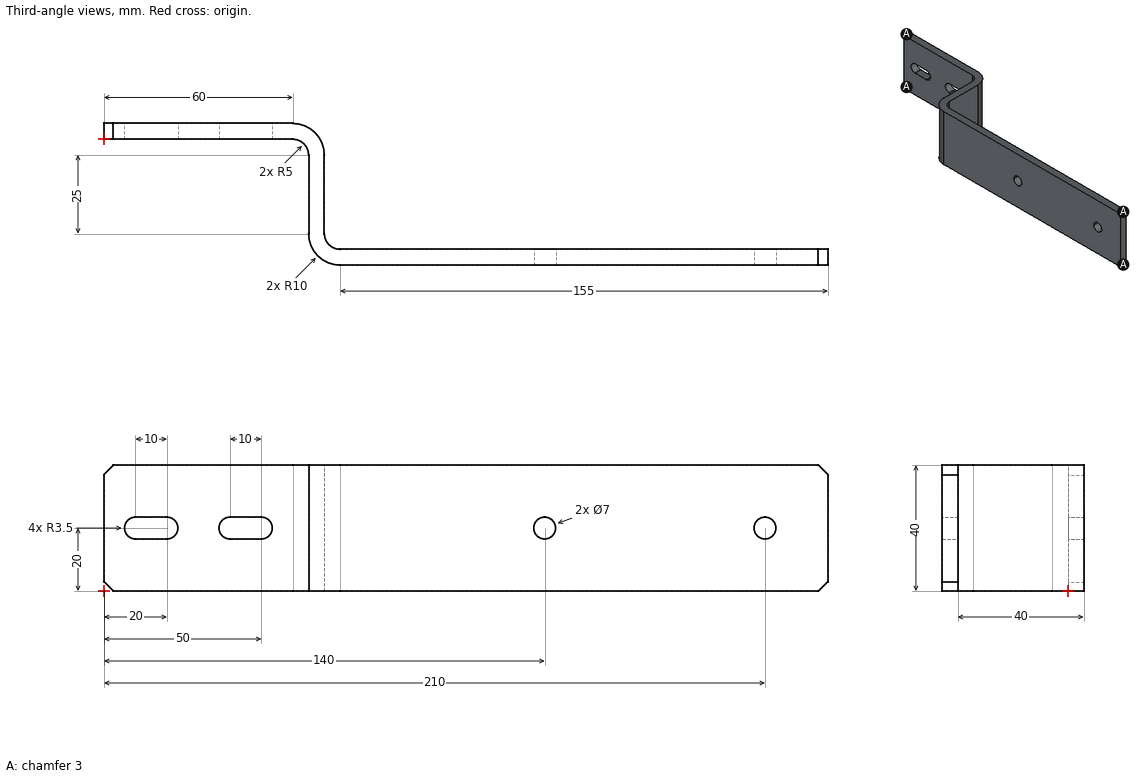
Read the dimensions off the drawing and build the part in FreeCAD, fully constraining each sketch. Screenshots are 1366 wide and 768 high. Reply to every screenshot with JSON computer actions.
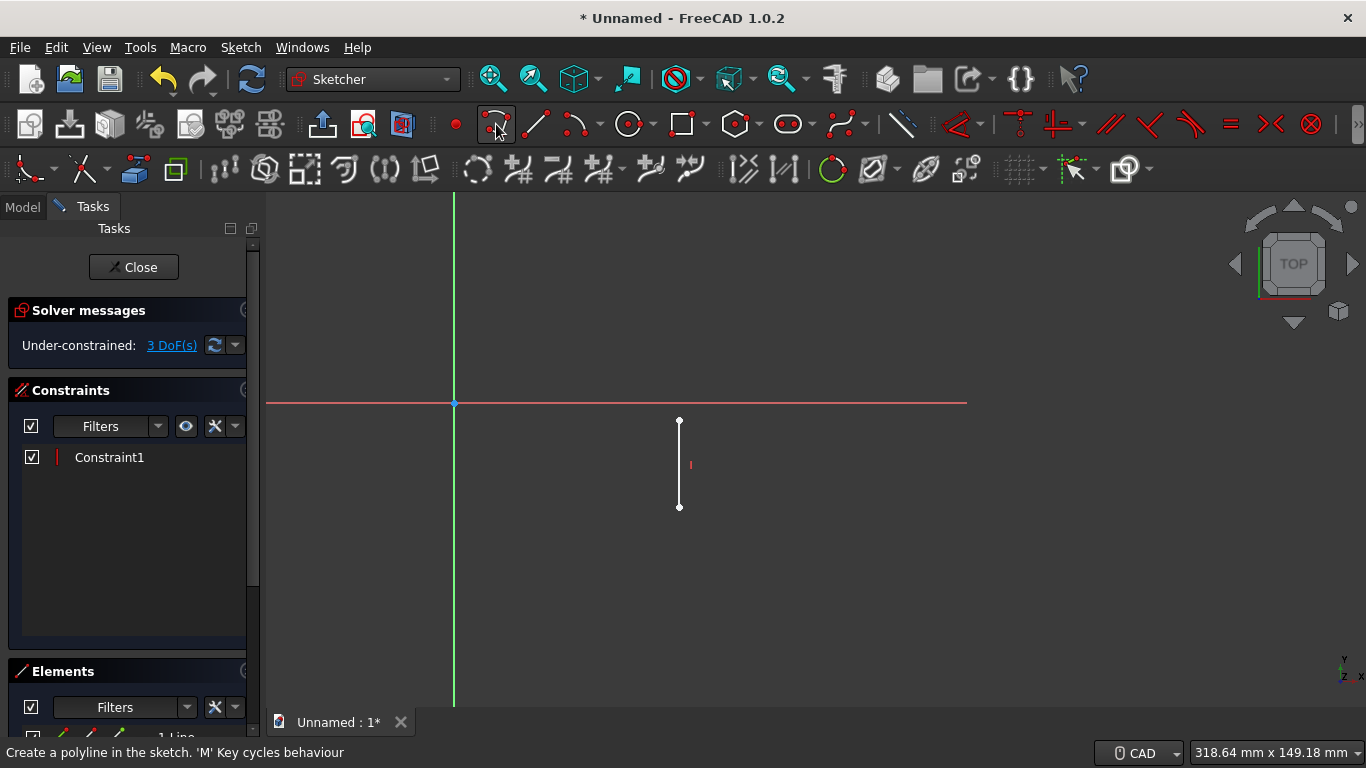
{"action": "left_click", "coordinate": [713, 541]}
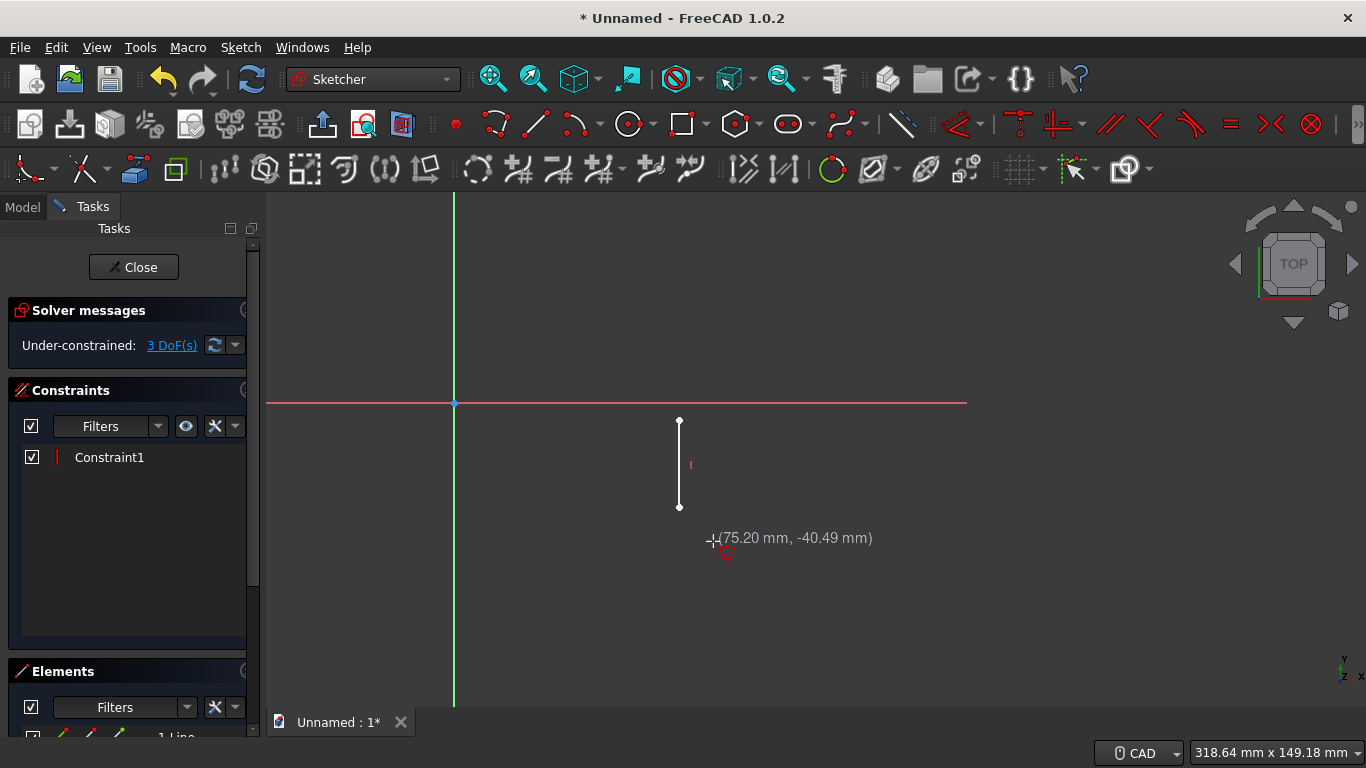
{"action": "scroll", "coordinate": [294, 386], "scroll_direction": "down", "scroll_amount": 1}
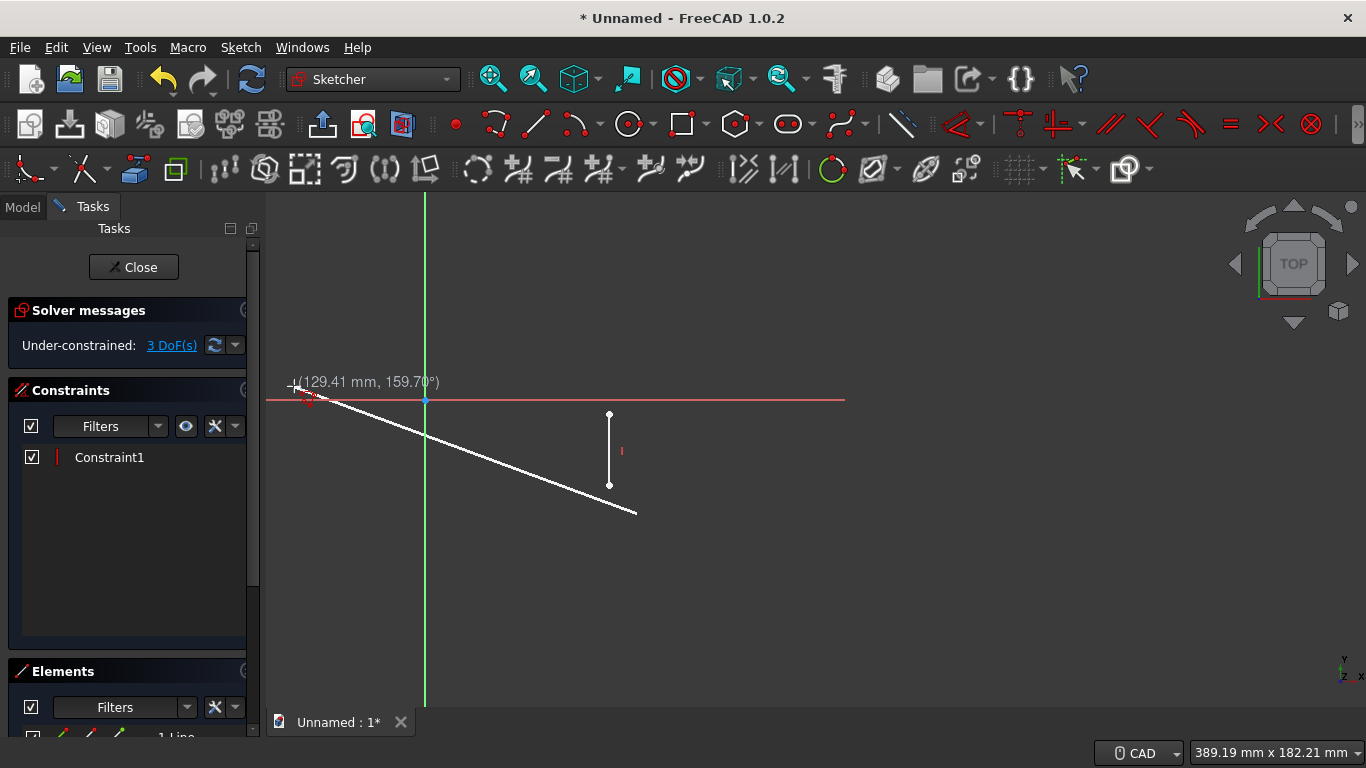
{"action": "left_click", "coordinate": [1075, 513]}
{"action": "left_click", "coordinate": [1075, 499]}
{"action": "left_click", "coordinate": [637, 499]}
{"action": "right_click", "coordinate": [637, 499]}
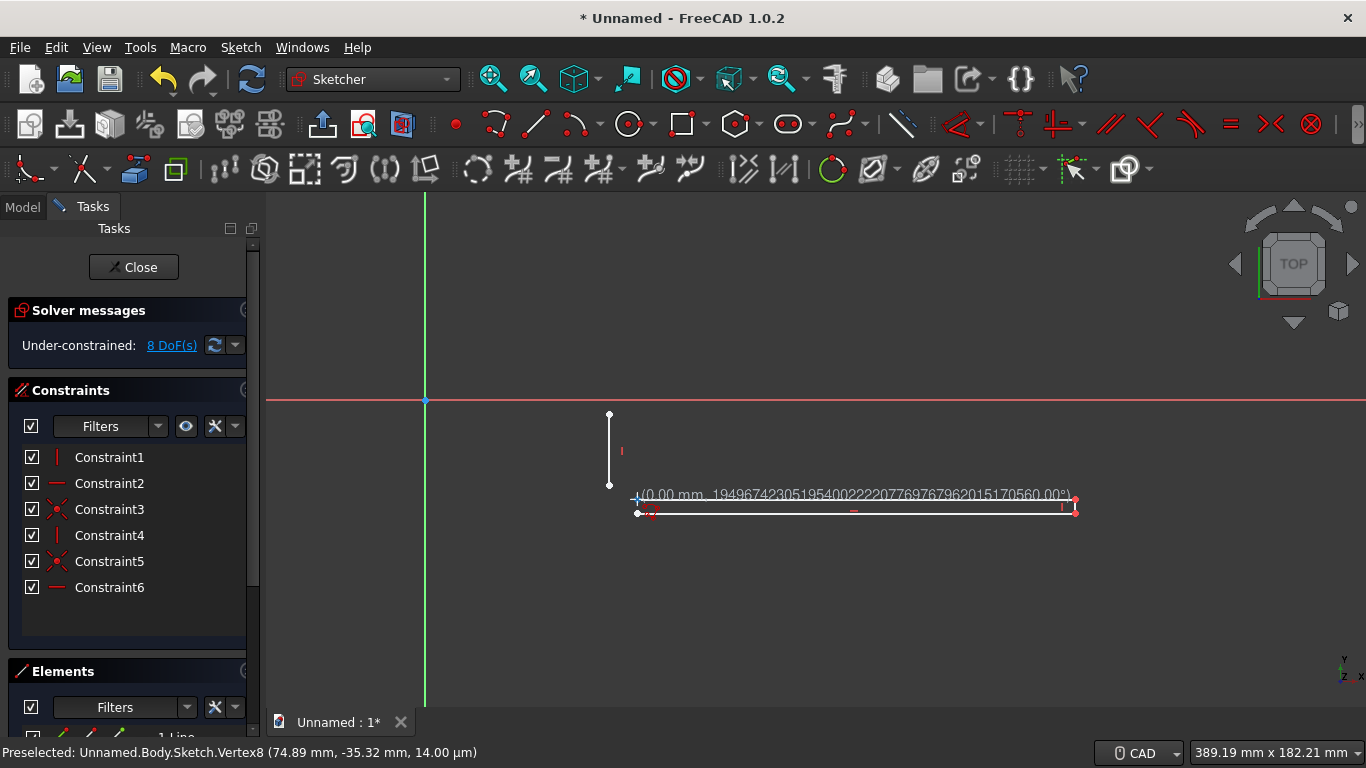
{"action": "left_click", "coordinate": [536, 124]}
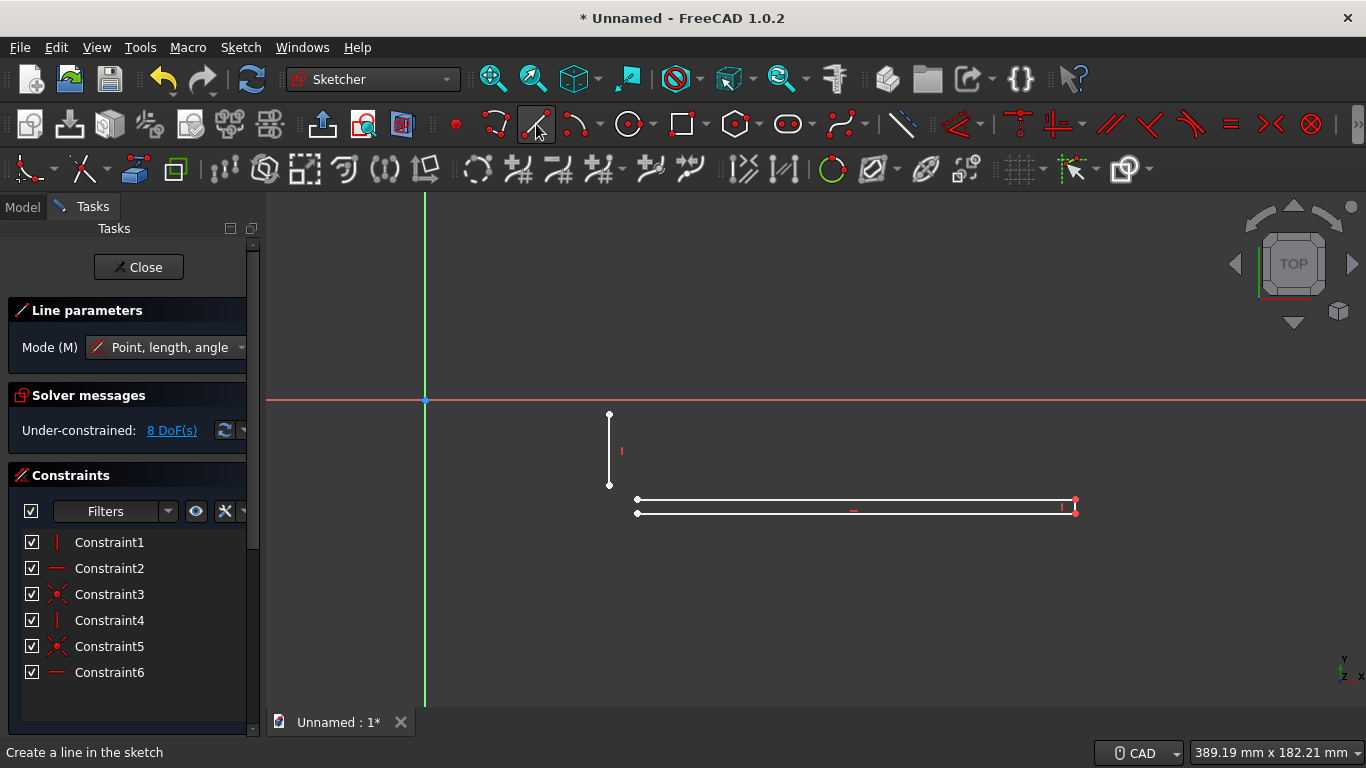
{"action": "left_click", "coordinate": [623, 485]}
{"action": "left_click", "coordinate": [623, 414]}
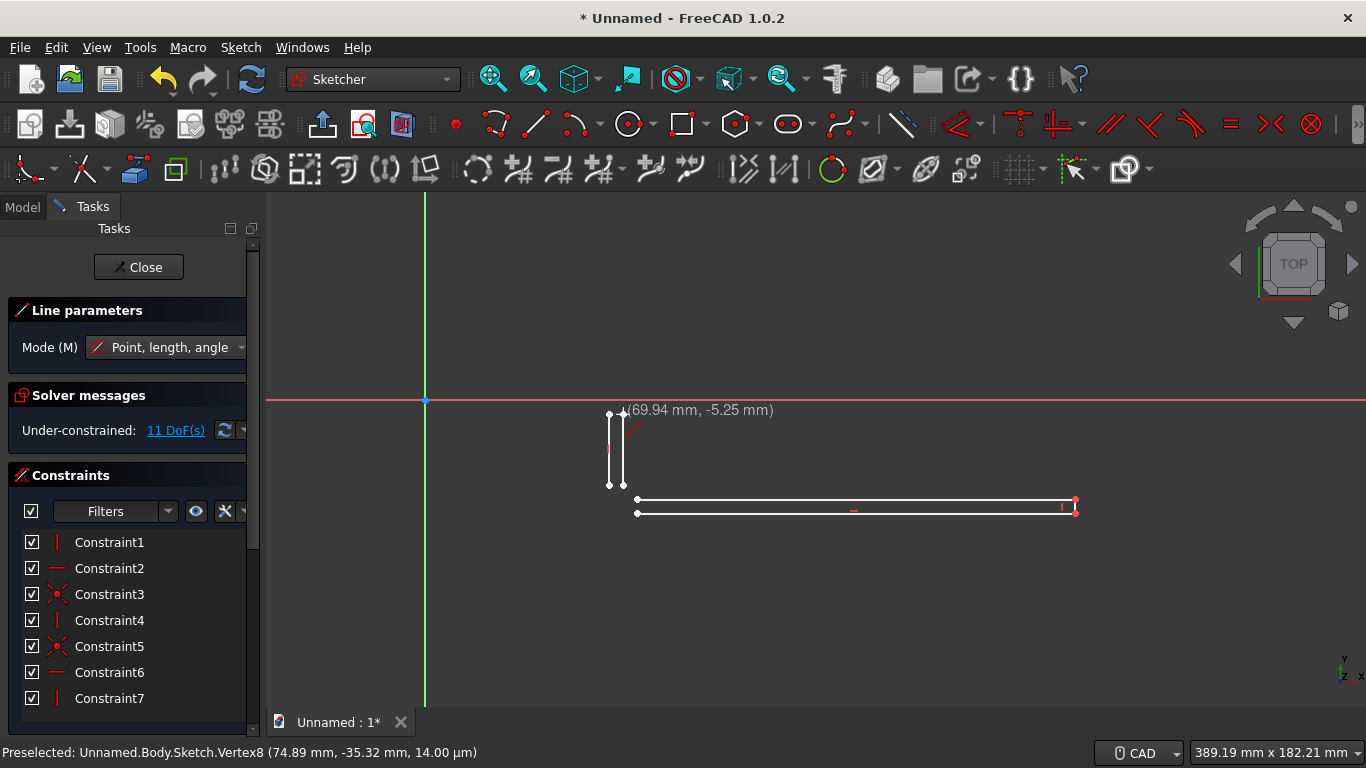
{"action": "left_click", "coordinate": [496, 124]}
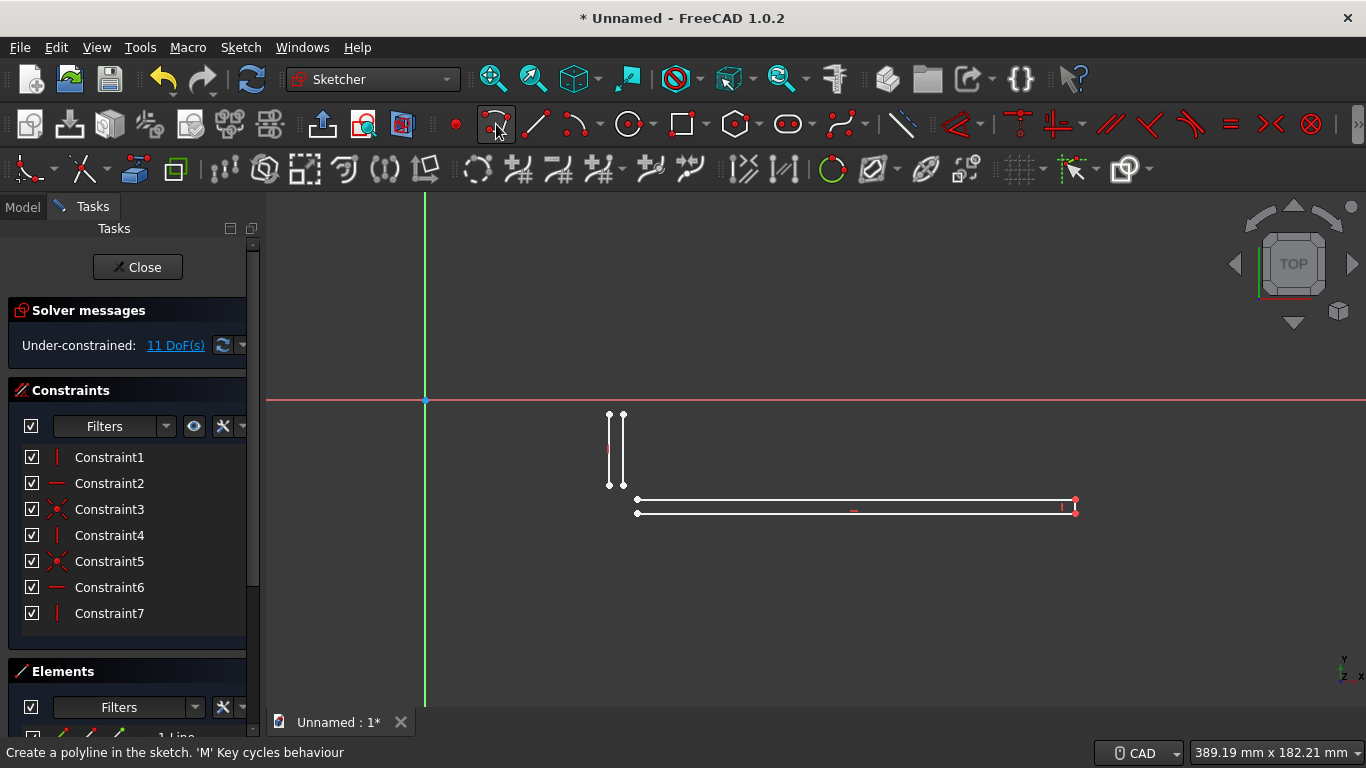
{"action": "left_click", "coordinate": [595, 386]}
{"action": "left_click", "coordinate": [425, 386]}
{"action": "left_click", "coordinate": [425, 400]}
{"action": "left_click", "coordinate": [595, 409]}
{"action": "right_click", "coordinate": [595, 409]}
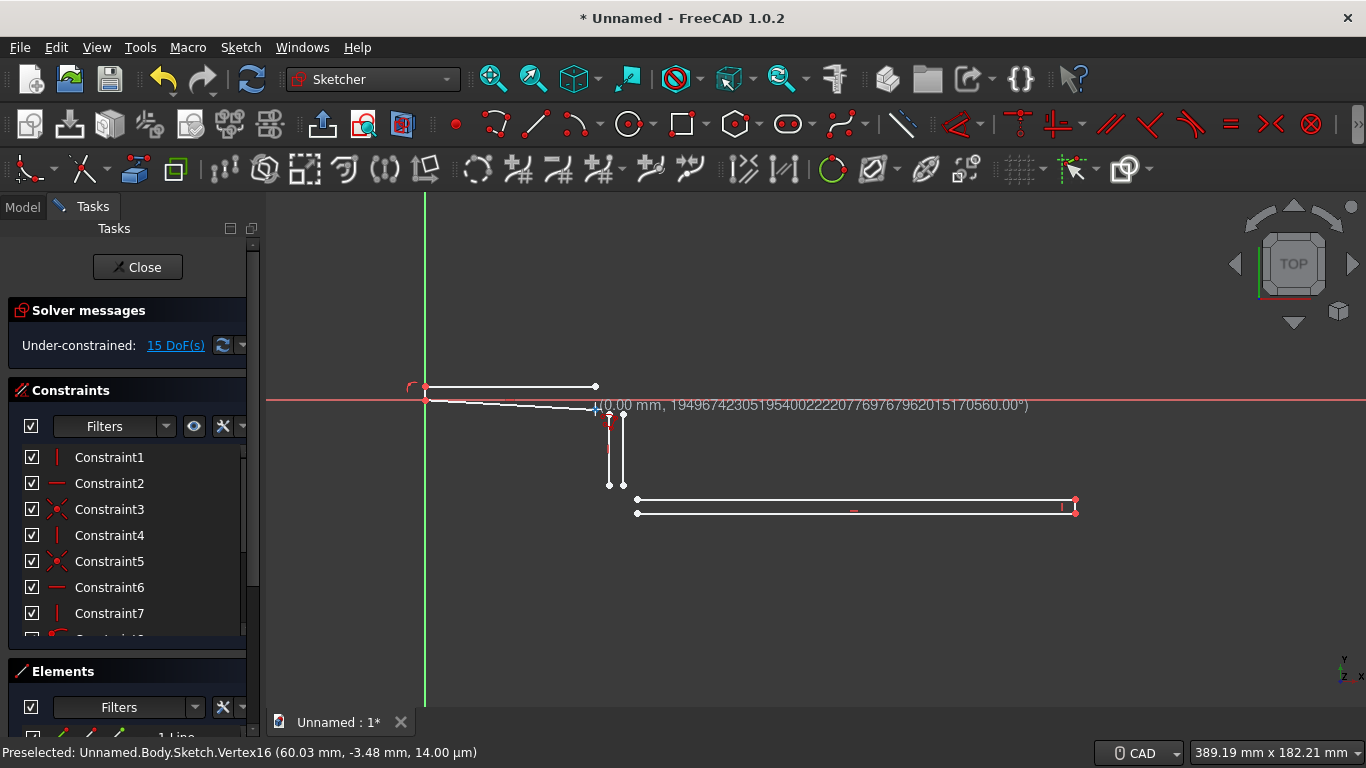
{"action": "left_click", "coordinate": [602, 124]}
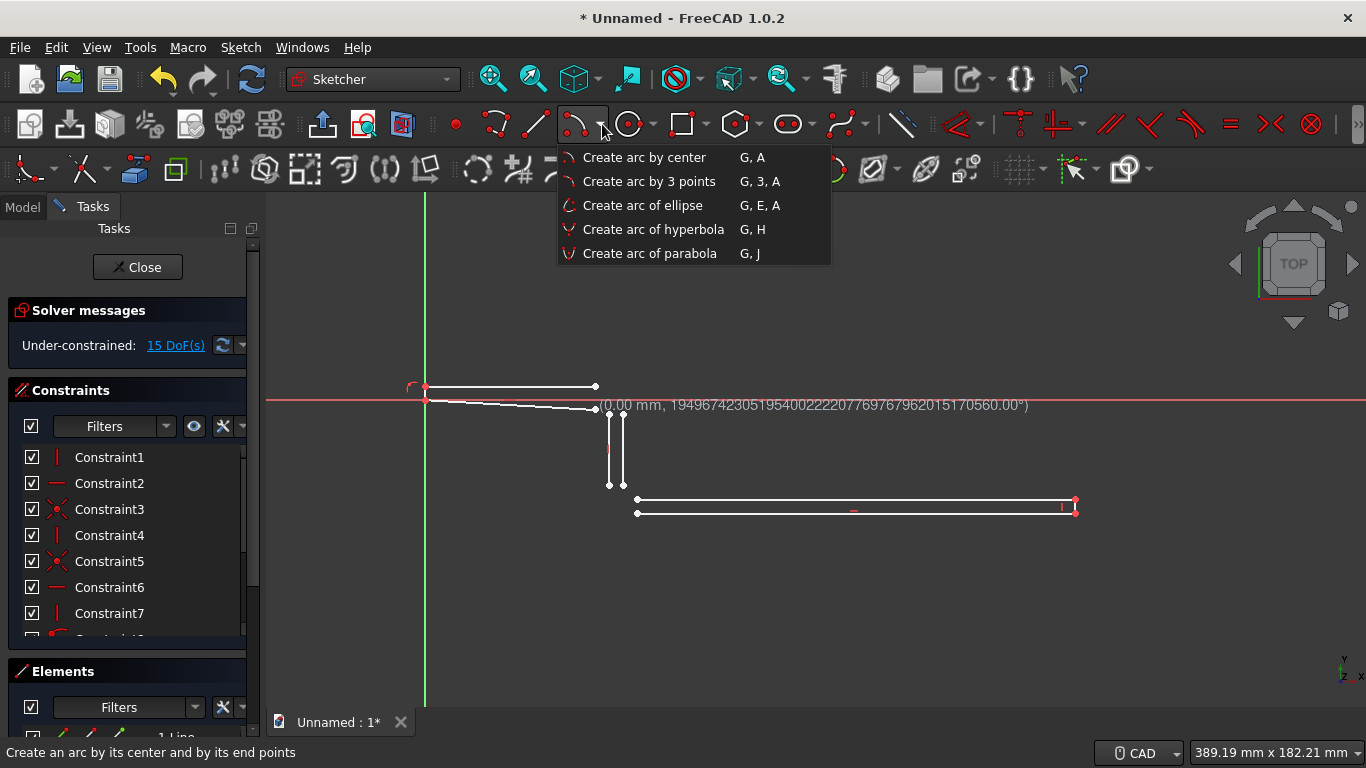
{"action": "left_click", "coordinate": [694, 181]}